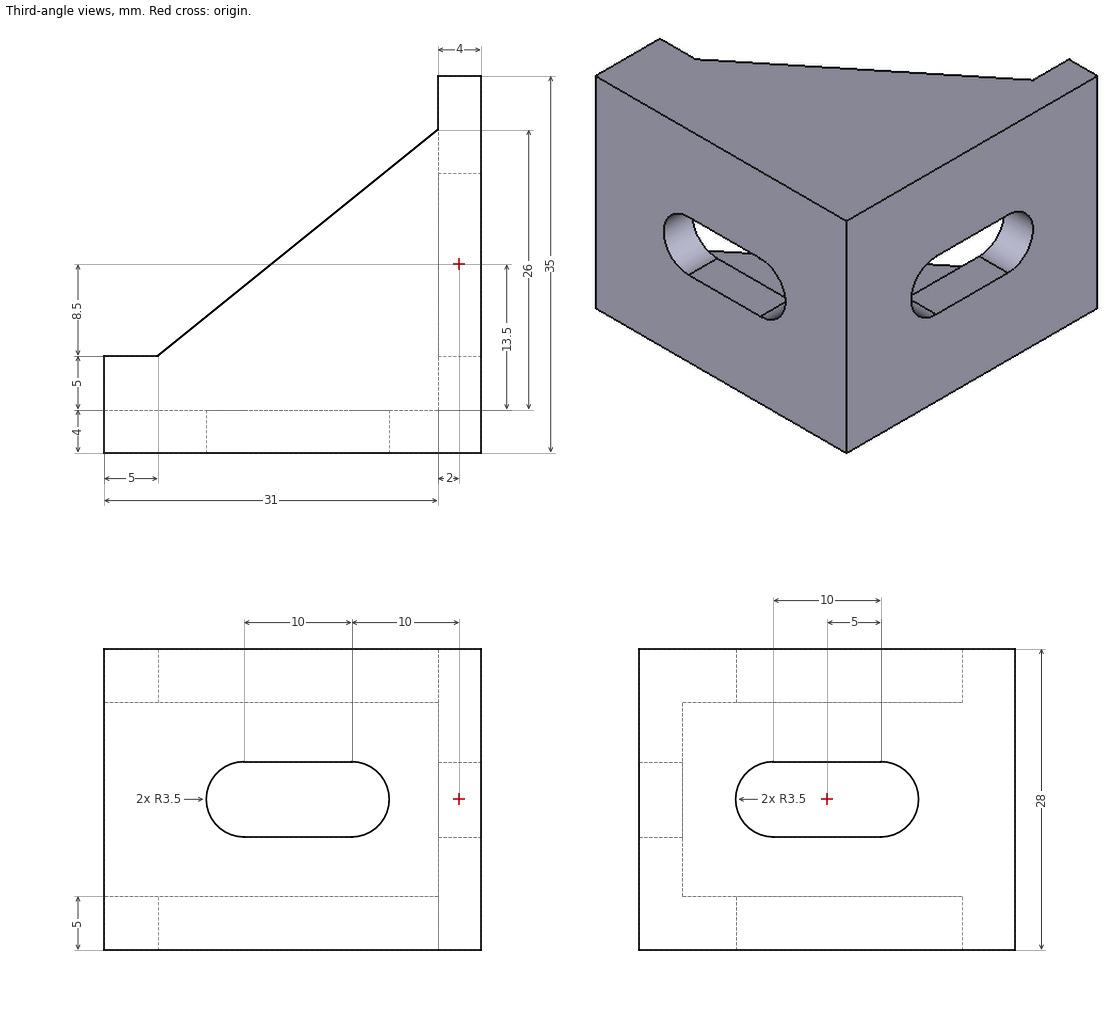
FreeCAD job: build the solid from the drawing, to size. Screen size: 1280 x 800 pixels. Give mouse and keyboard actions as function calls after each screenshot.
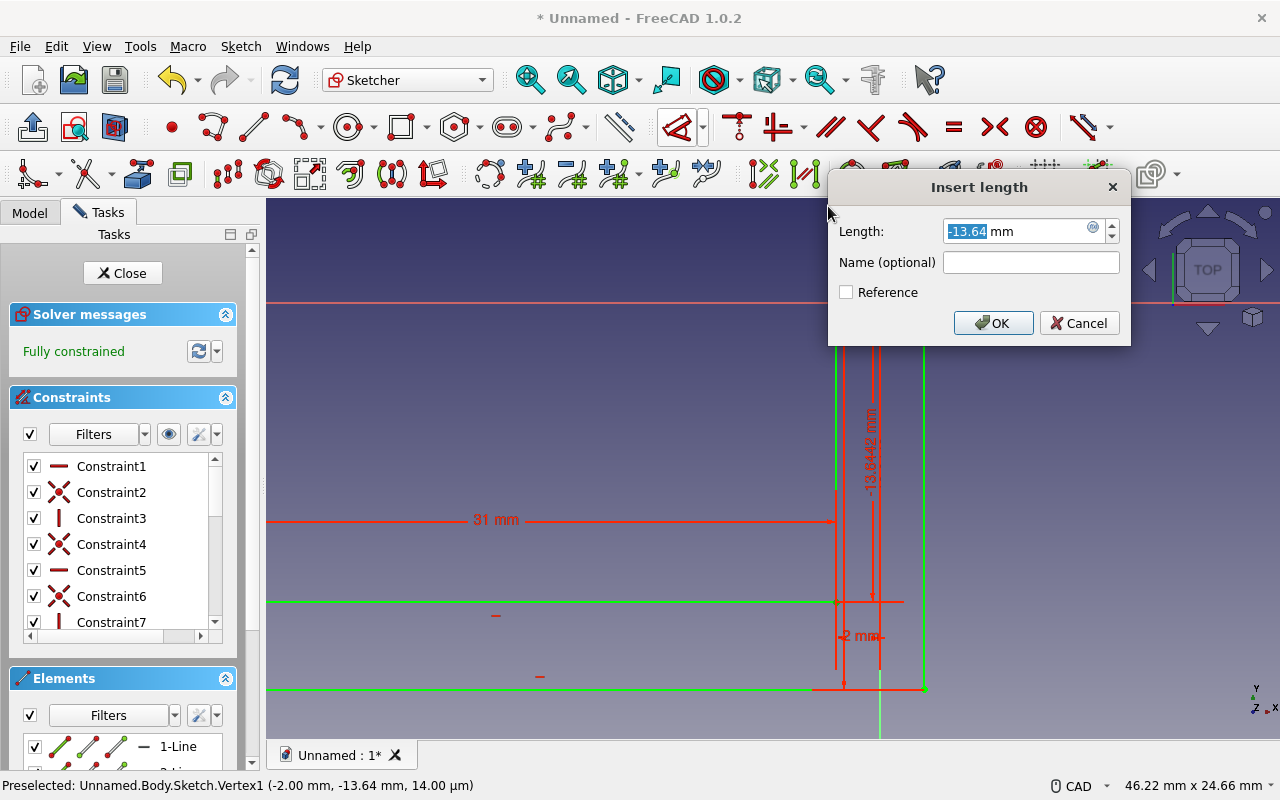
text(-13.5)
key(Return)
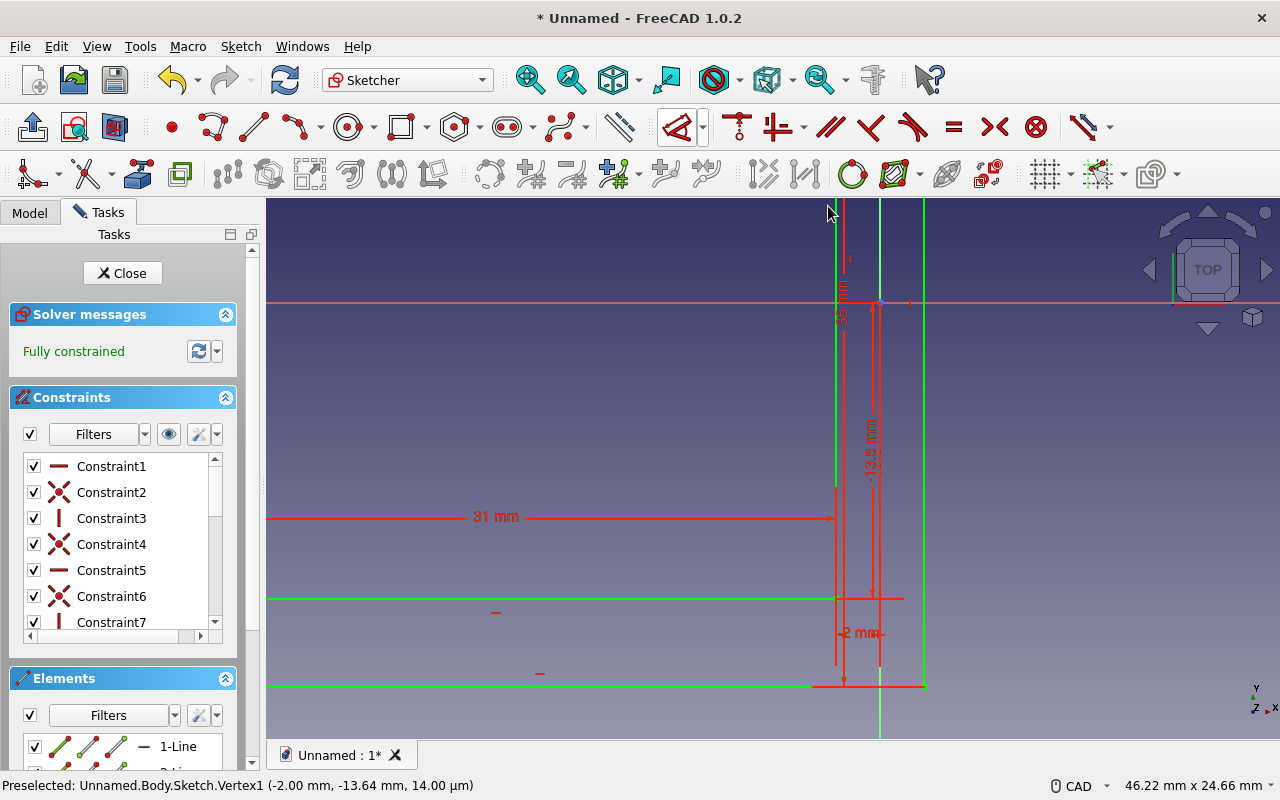
click(123, 273)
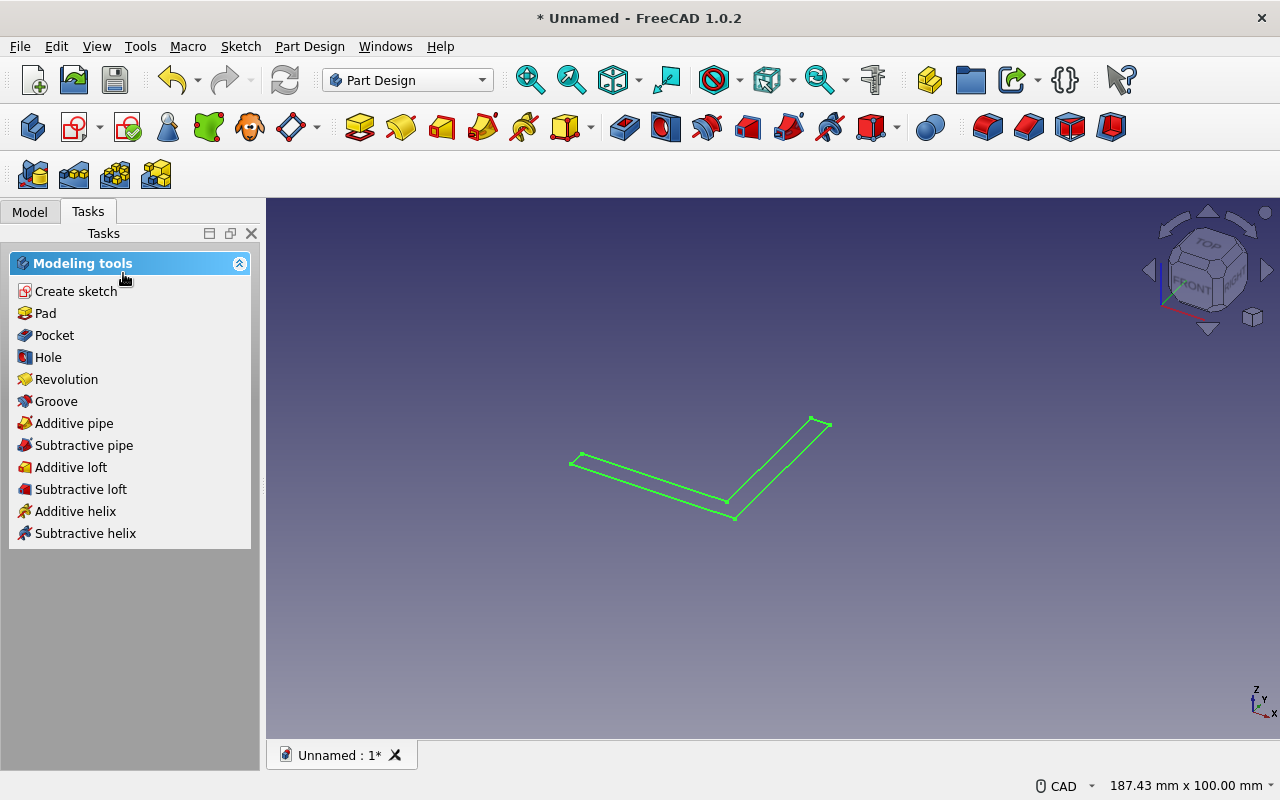
click(360, 128)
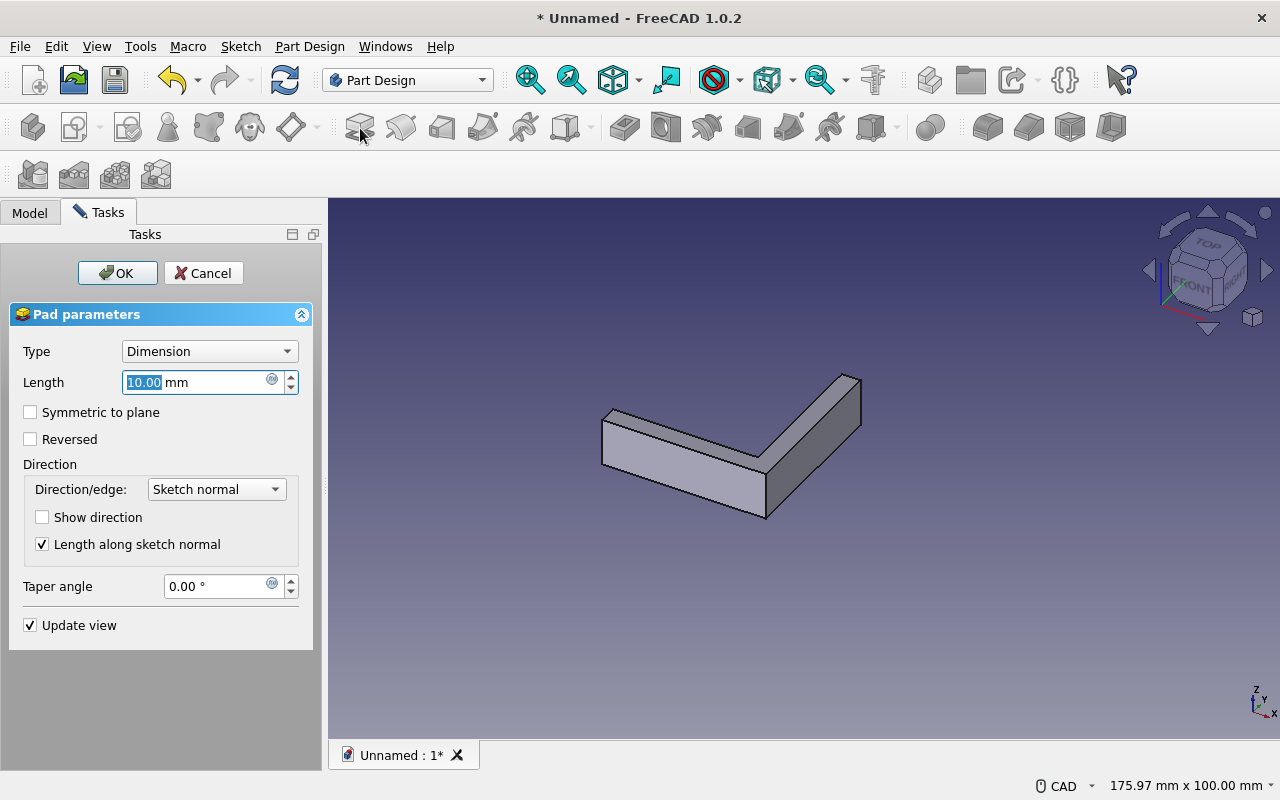
text(28)
key(Tab)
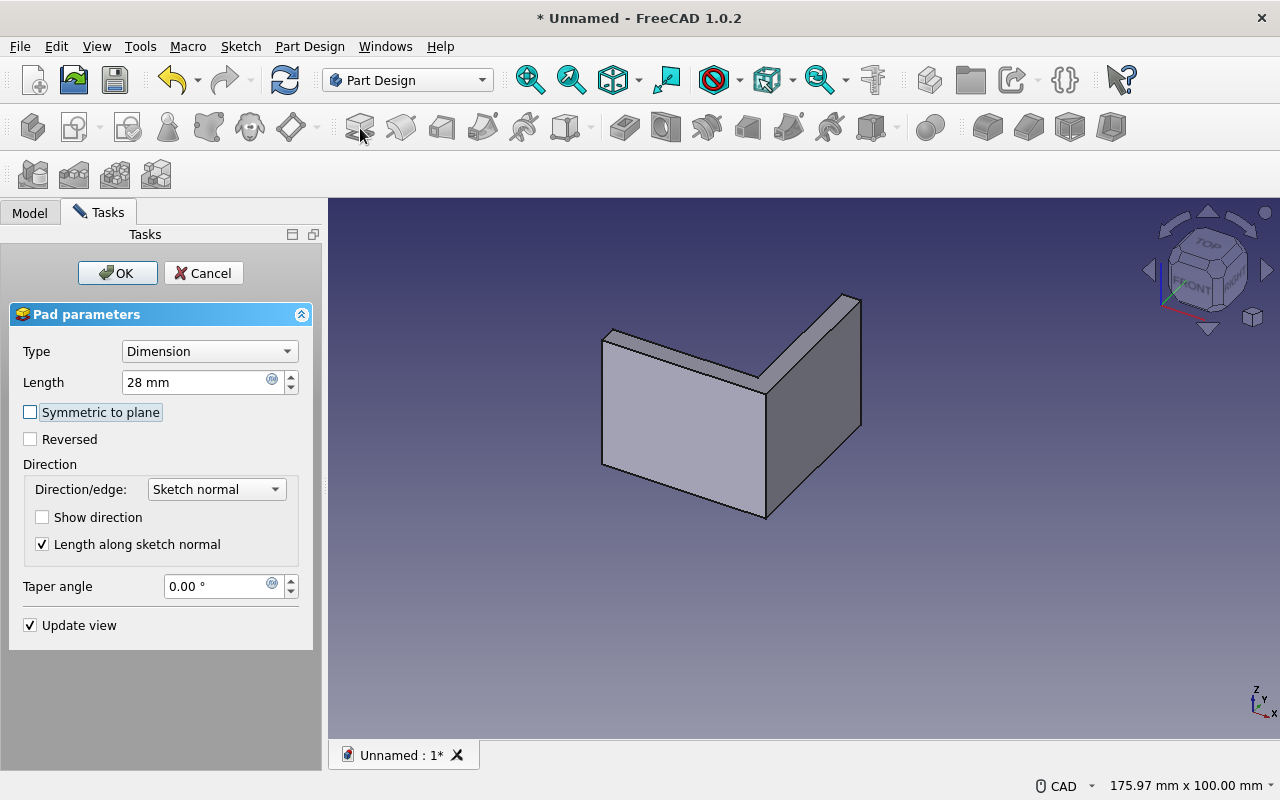
click(31, 412)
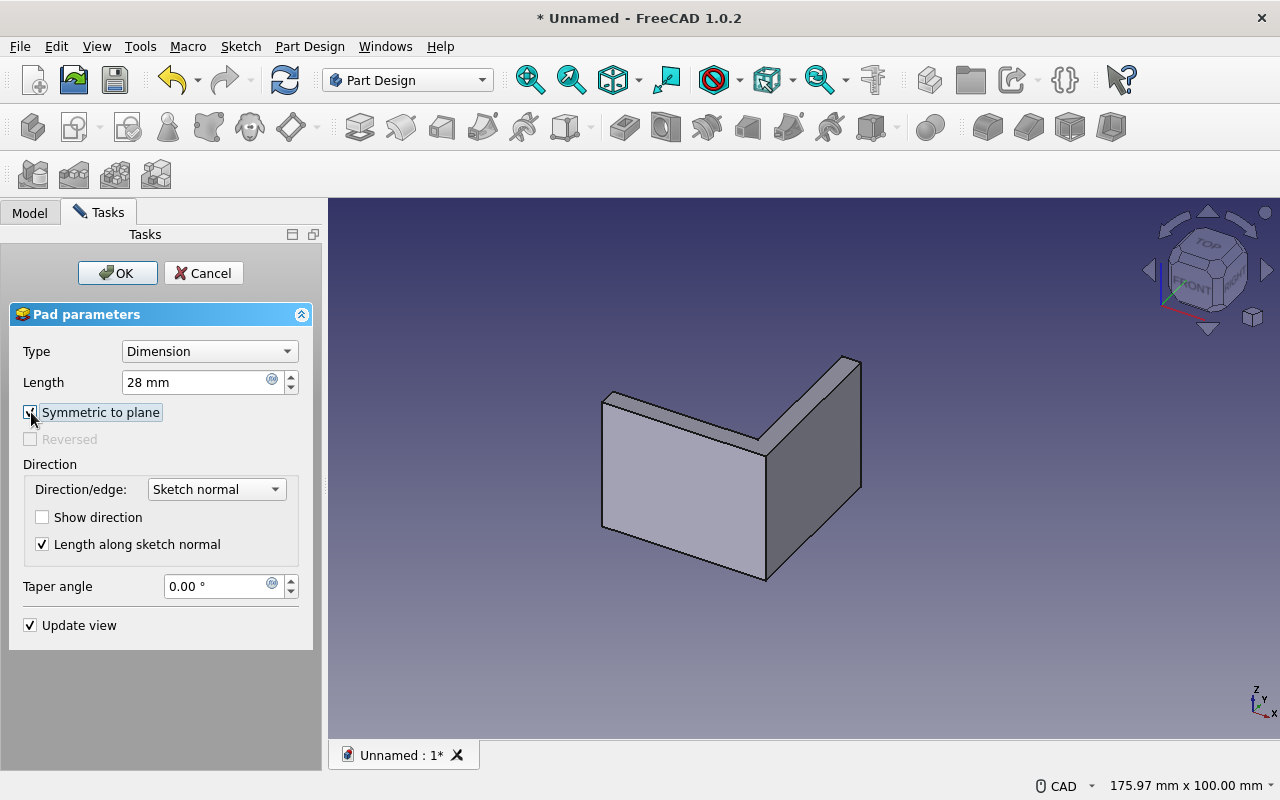
click(118, 273)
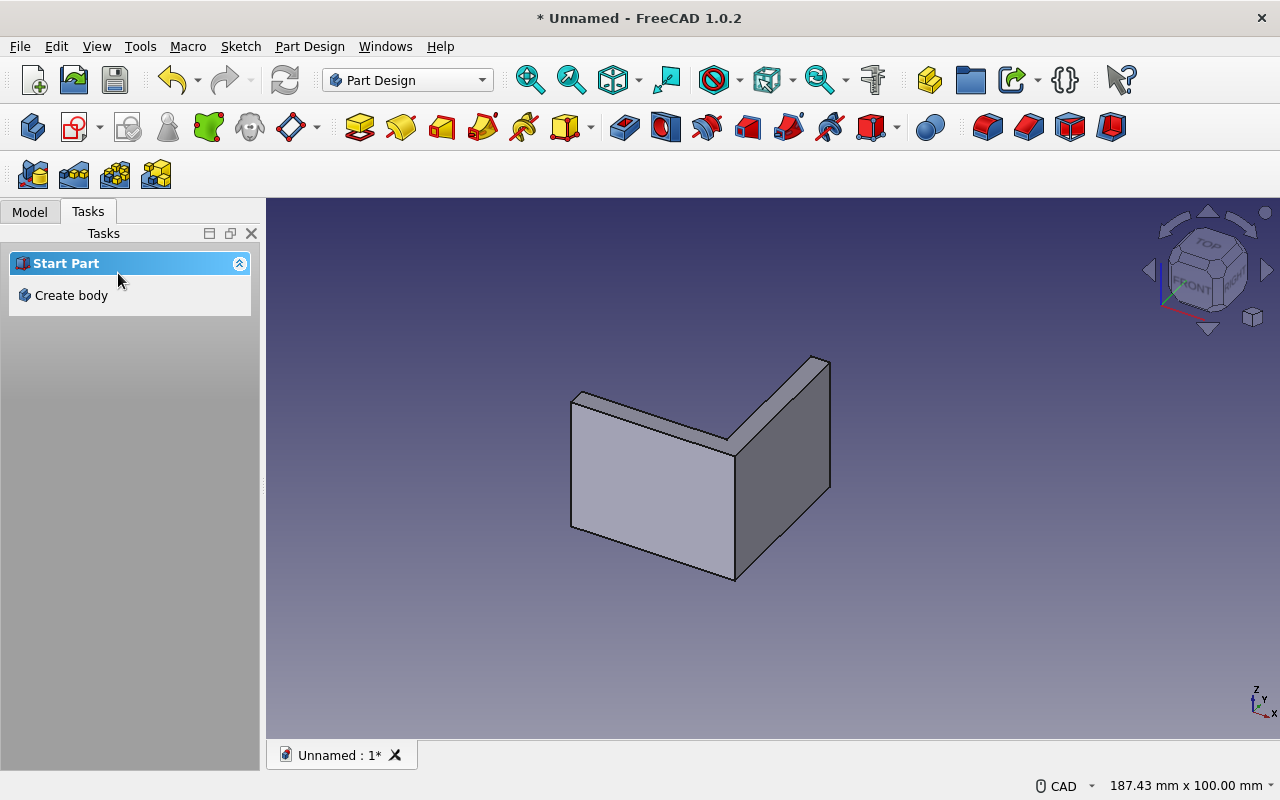
key(5)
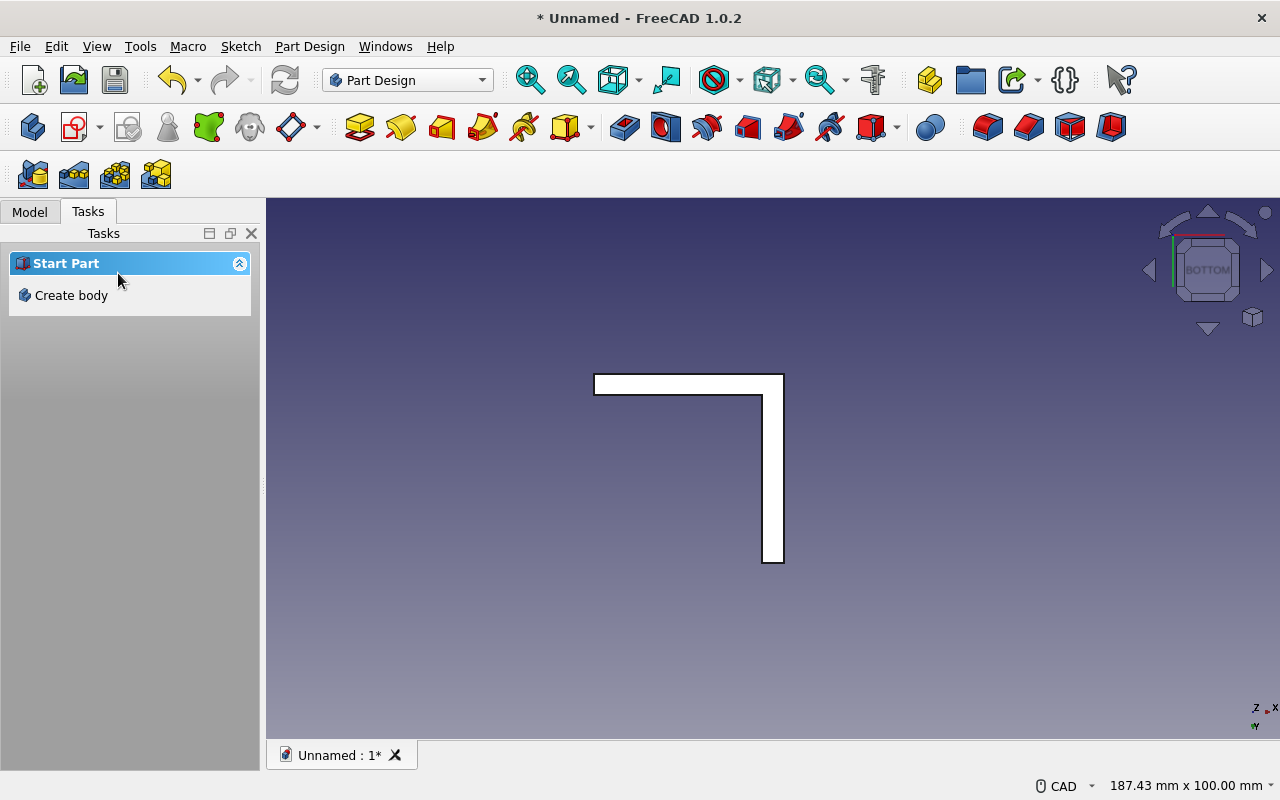
click(531, 80)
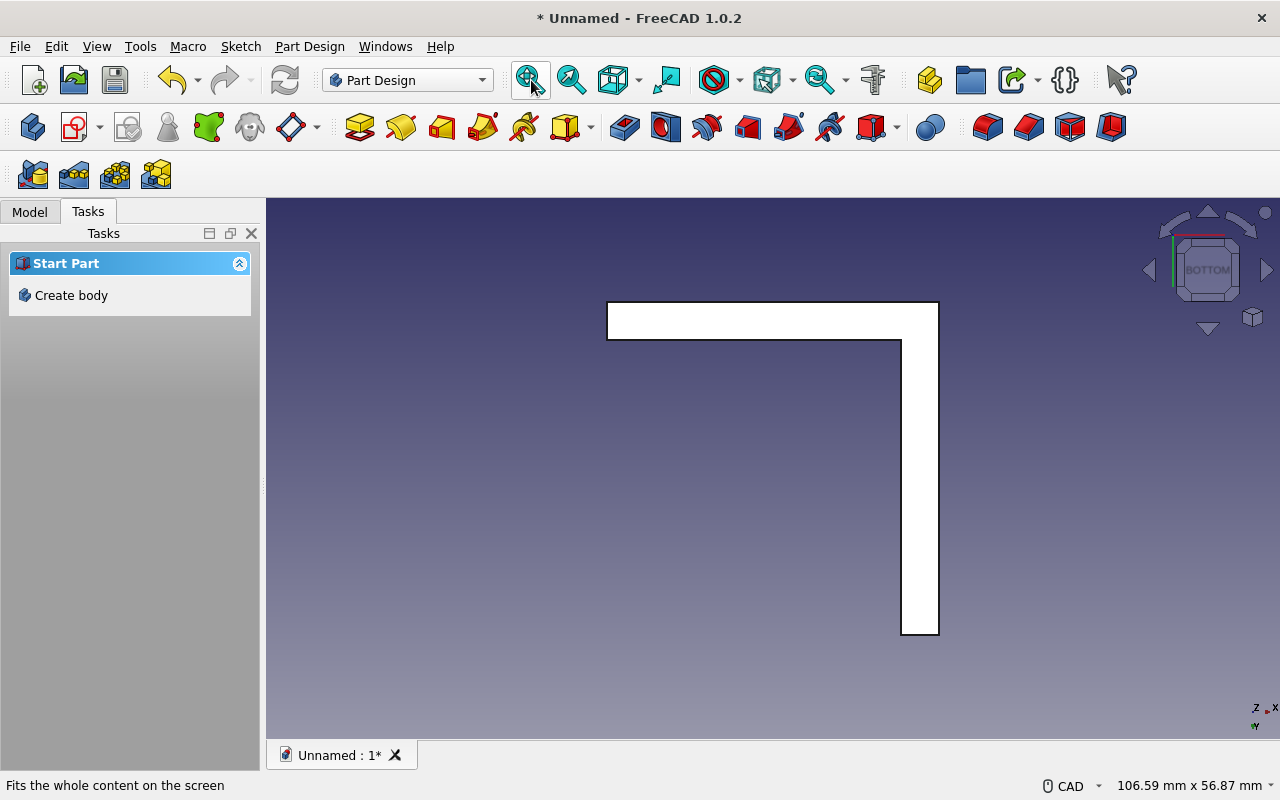
click(916, 325)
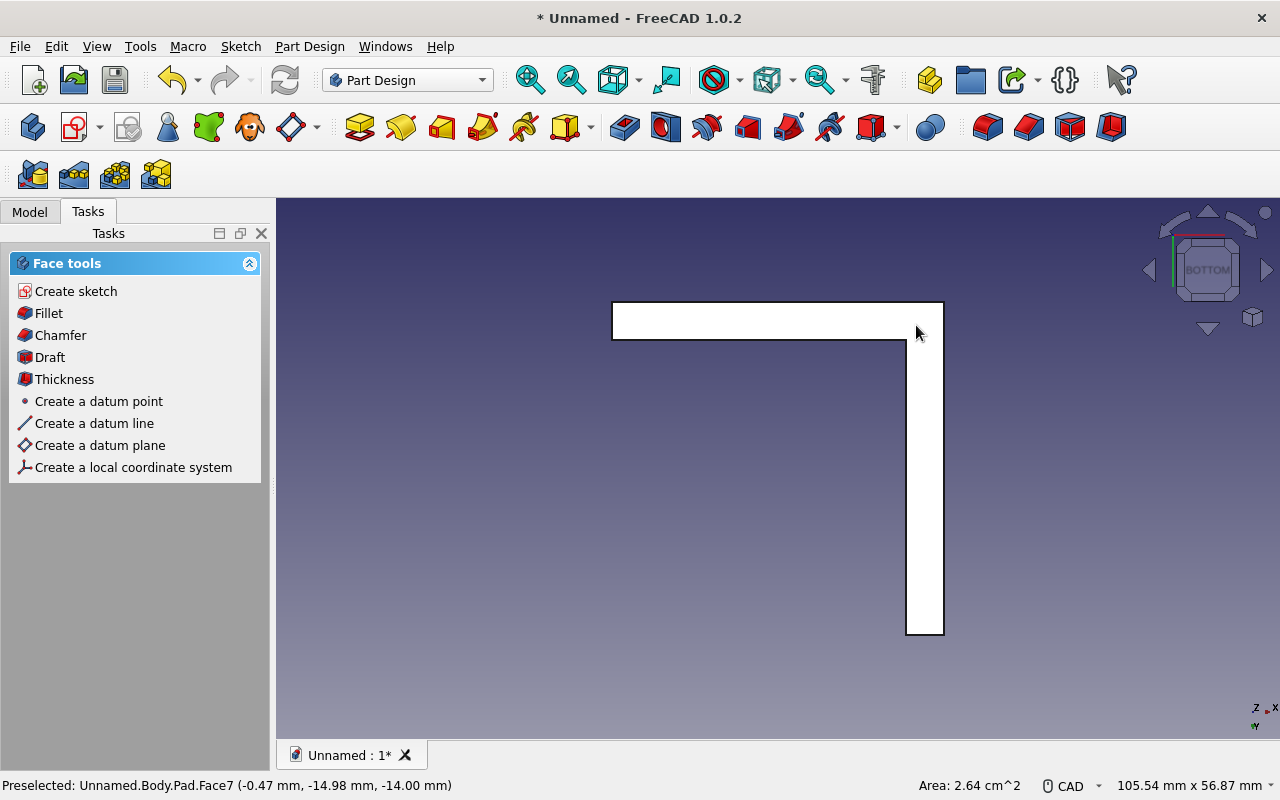
click(74, 128)